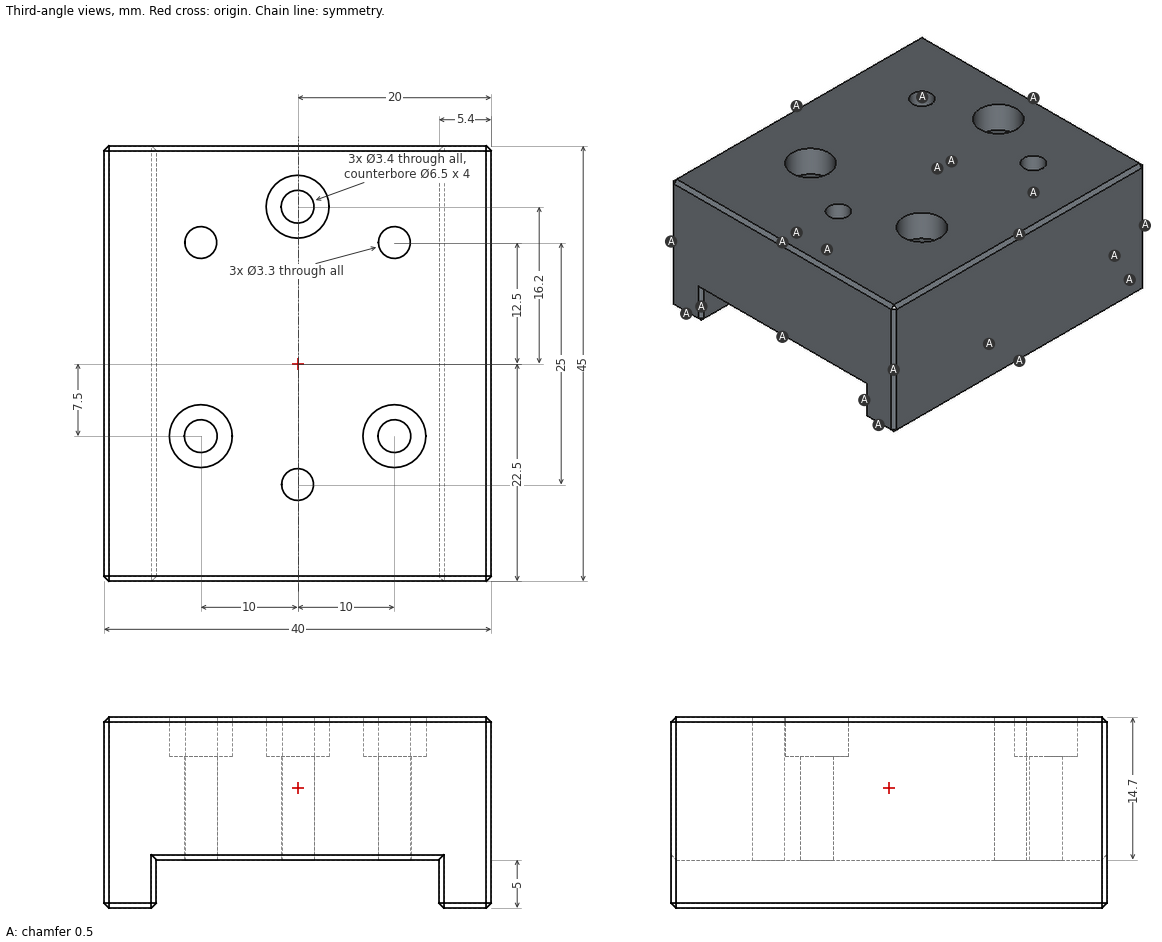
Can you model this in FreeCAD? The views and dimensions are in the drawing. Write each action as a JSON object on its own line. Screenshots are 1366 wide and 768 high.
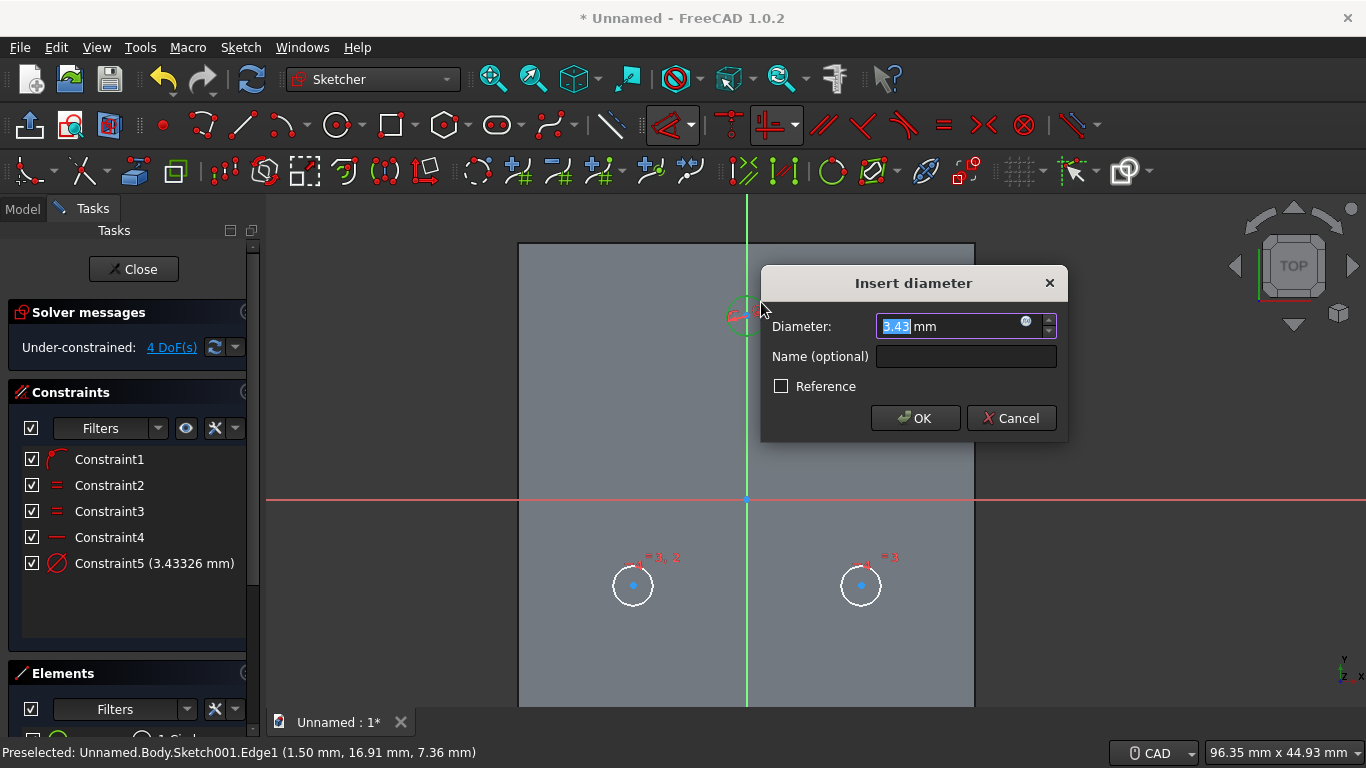
{"action": "type", "text": "3.4"}
{"action": "key", "text": "Return"}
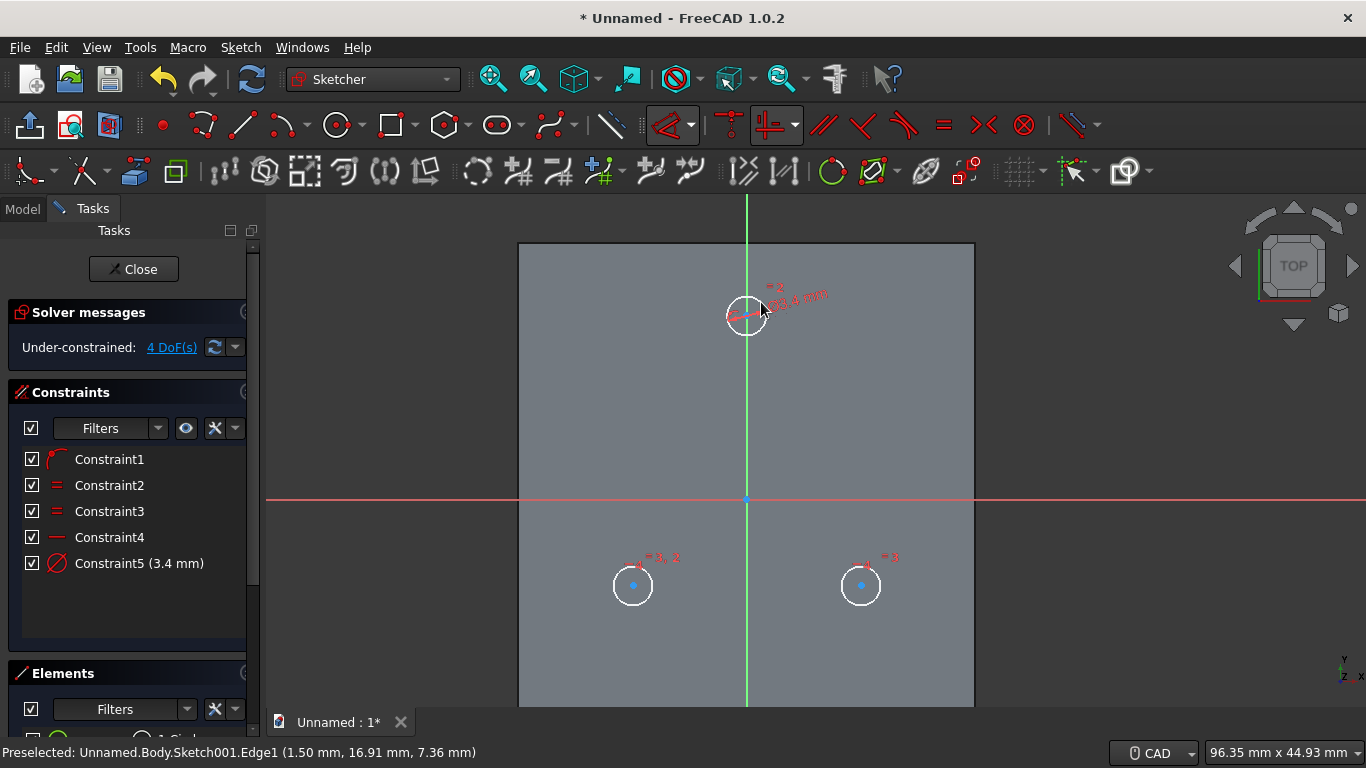
{"action": "left_click", "coordinate": [633, 586]}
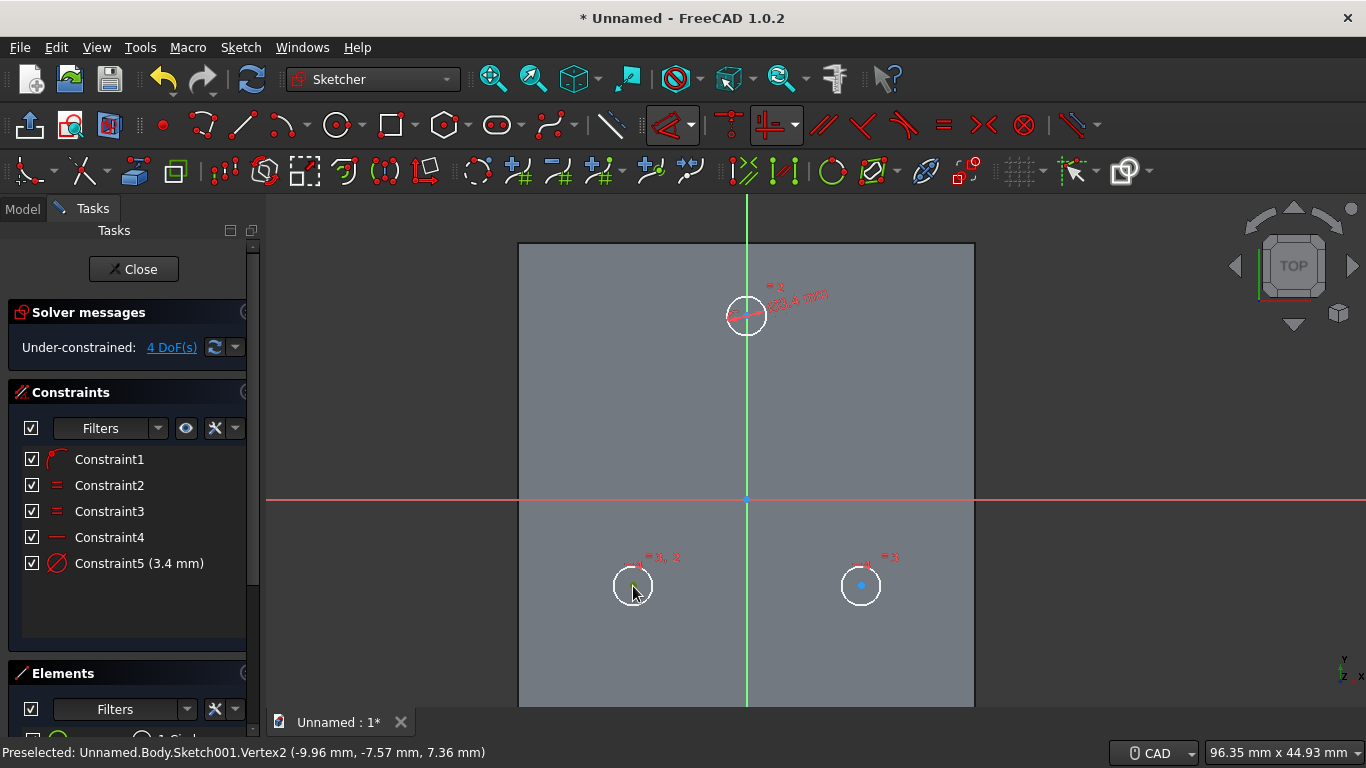
{"action": "key", "text": "l"}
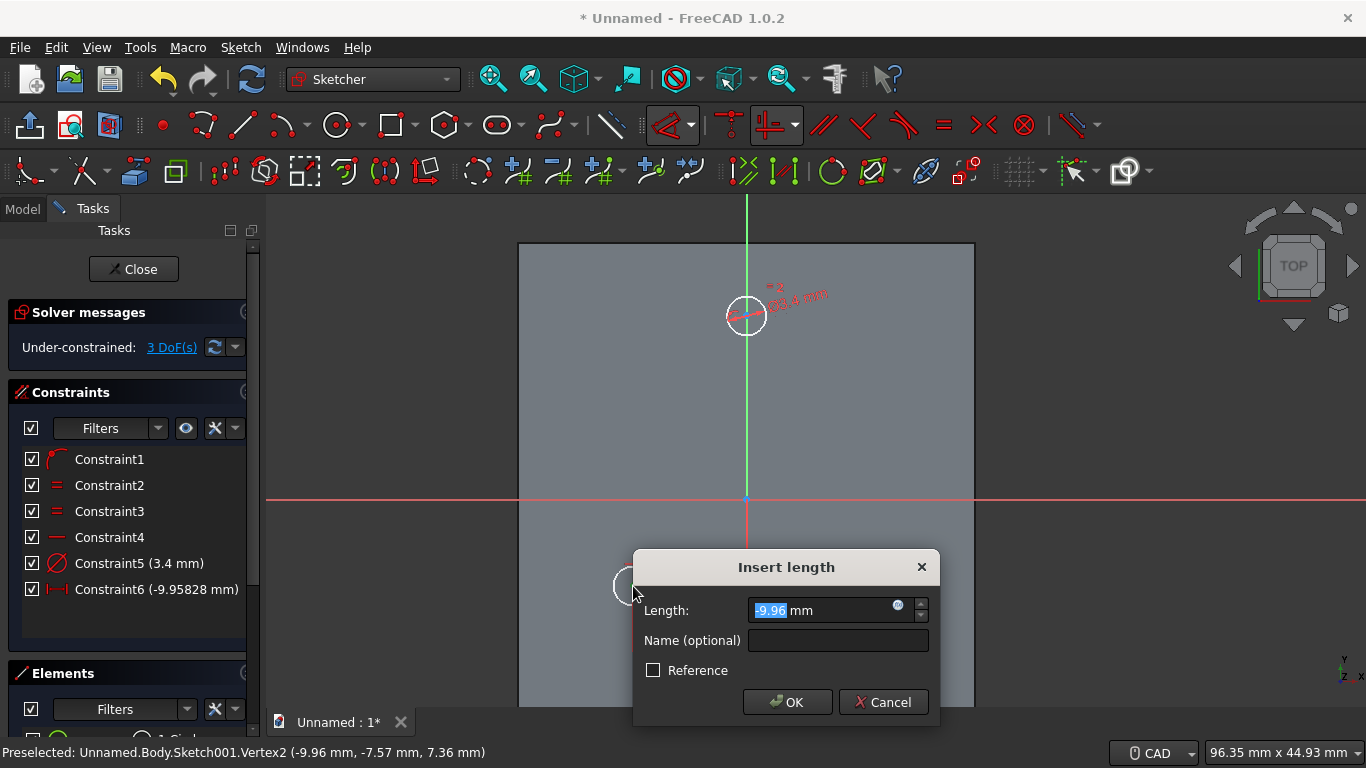
{"action": "type", "text": "-10"}
{"action": "key", "text": "Return"}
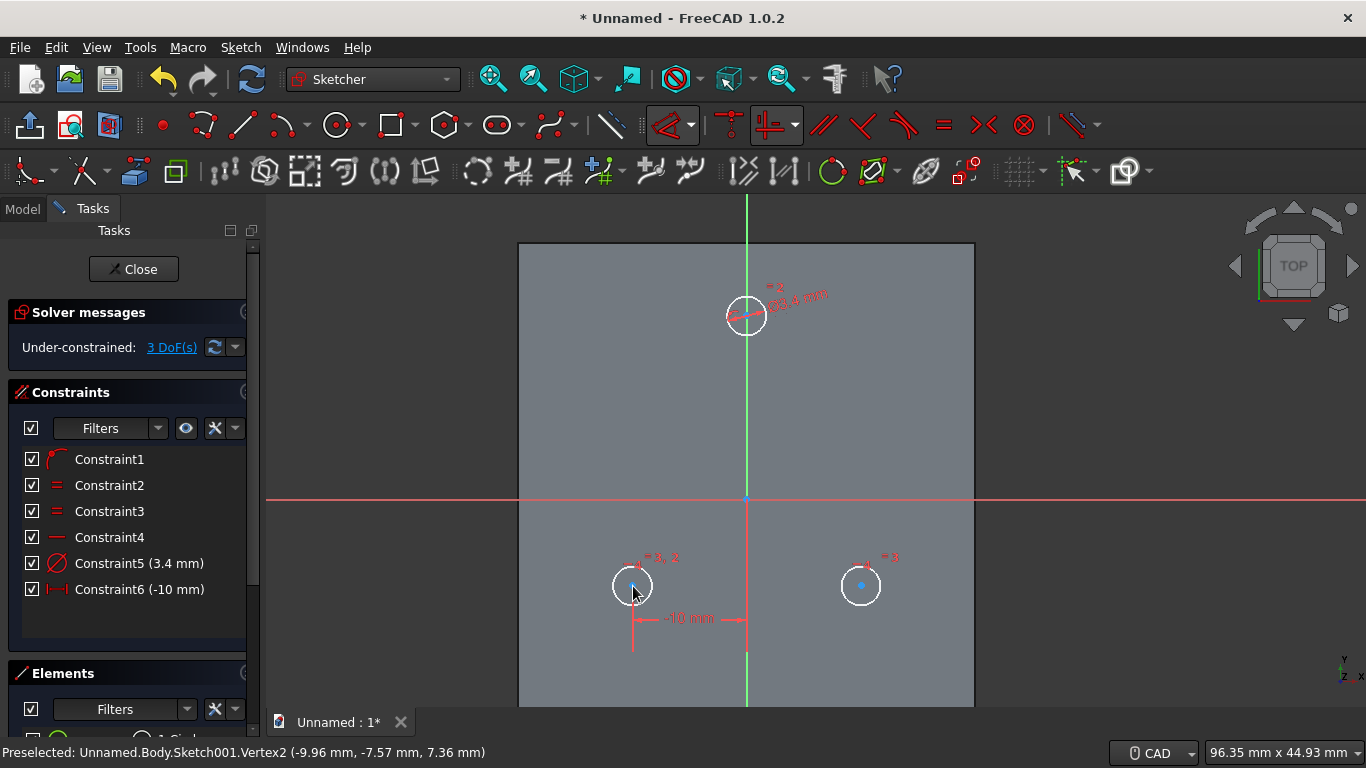
{"action": "left_click", "coordinate": [861, 586]}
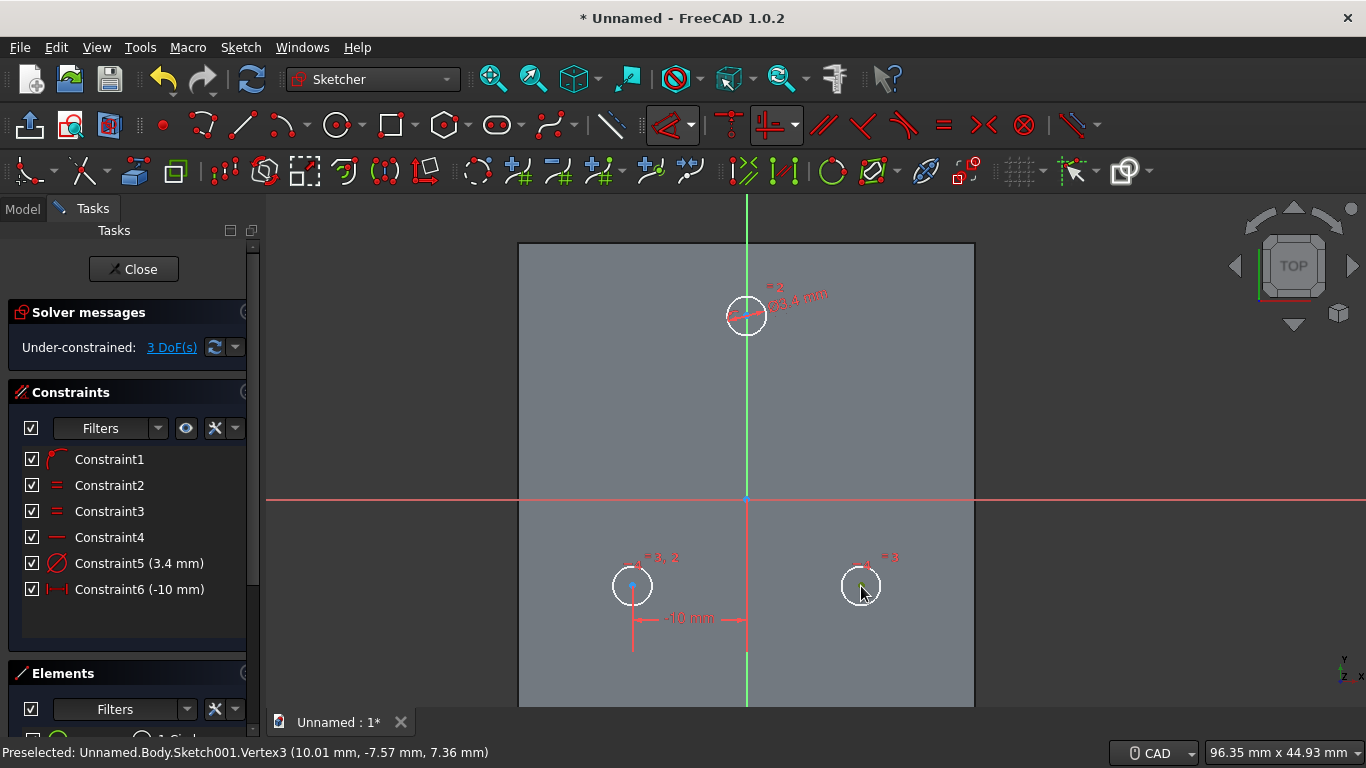
{"action": "left_click", "coordinate": [694, 126]}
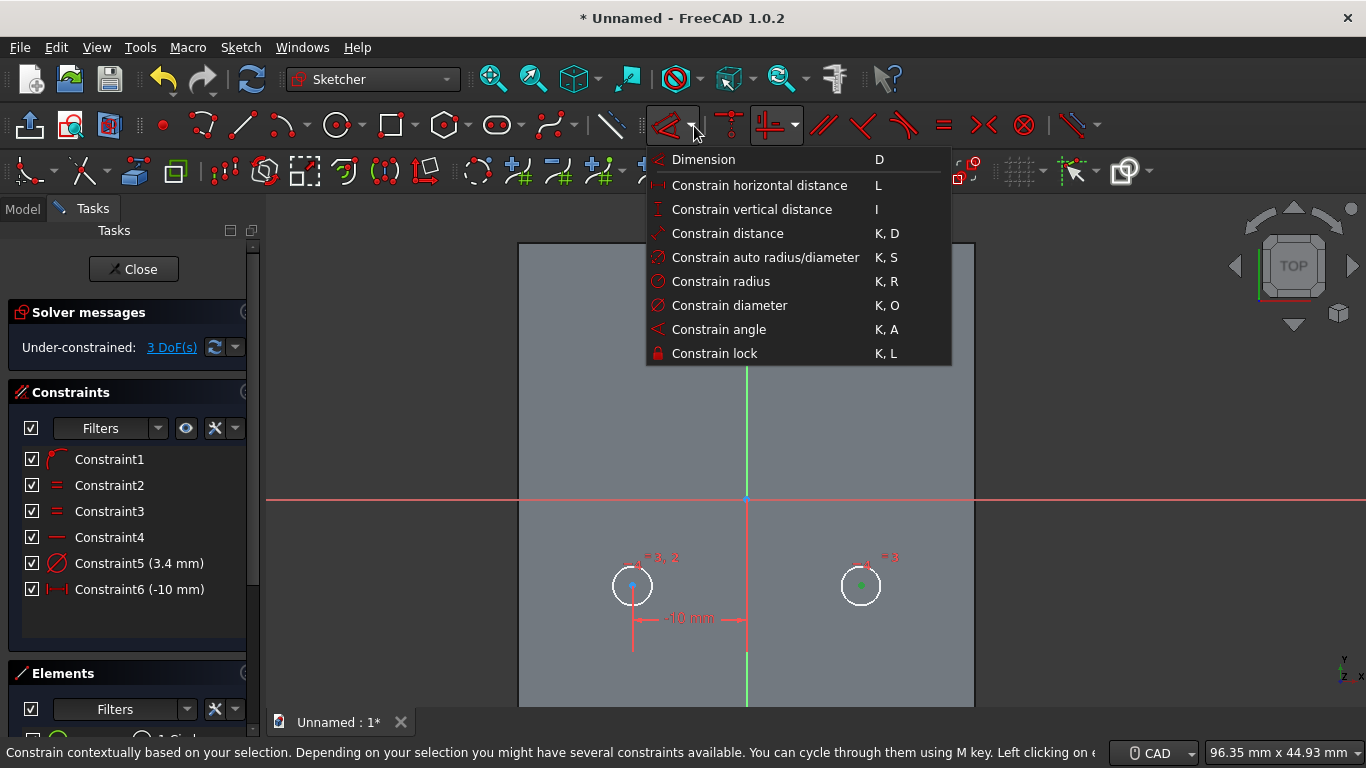
{"action": "left_click", "coordinate": [799, 185]}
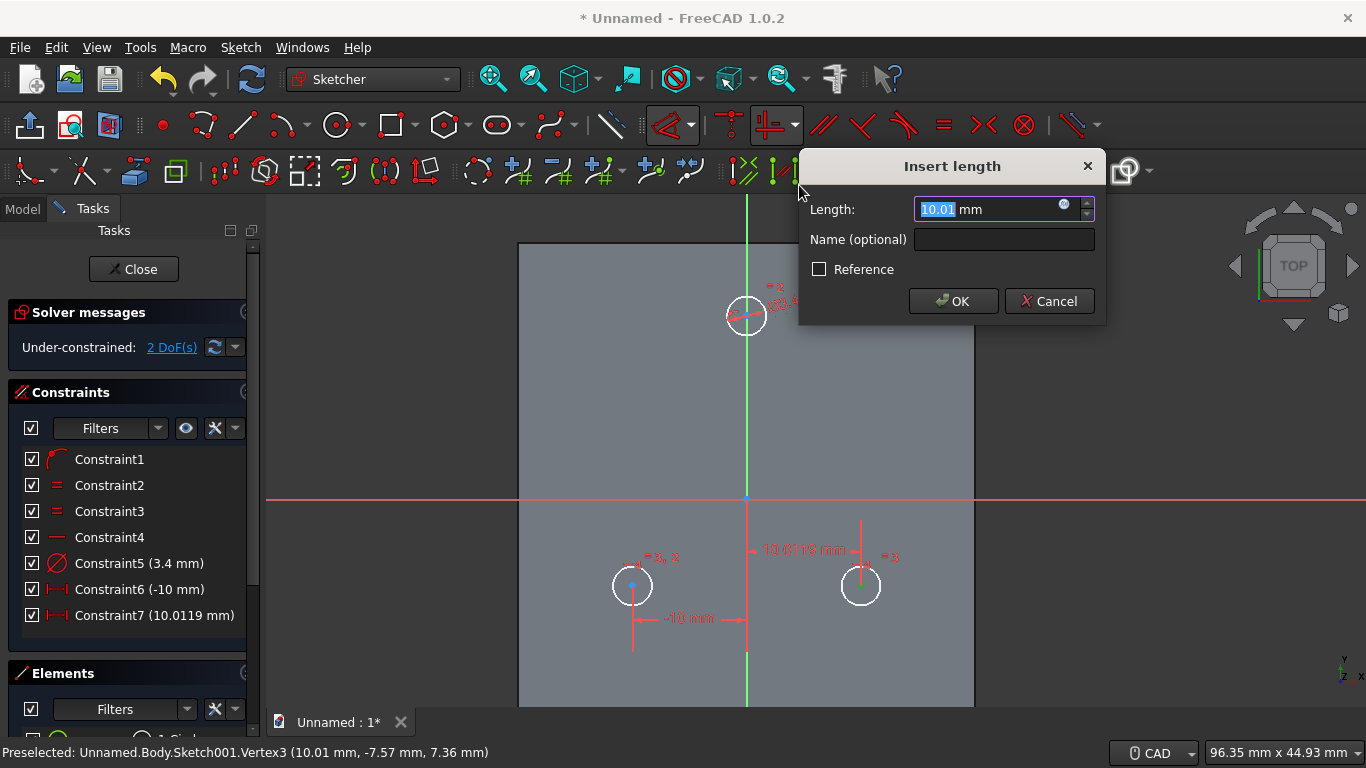
{"action": "type", "text": "10"}
{"action": "key", "text": "Return"}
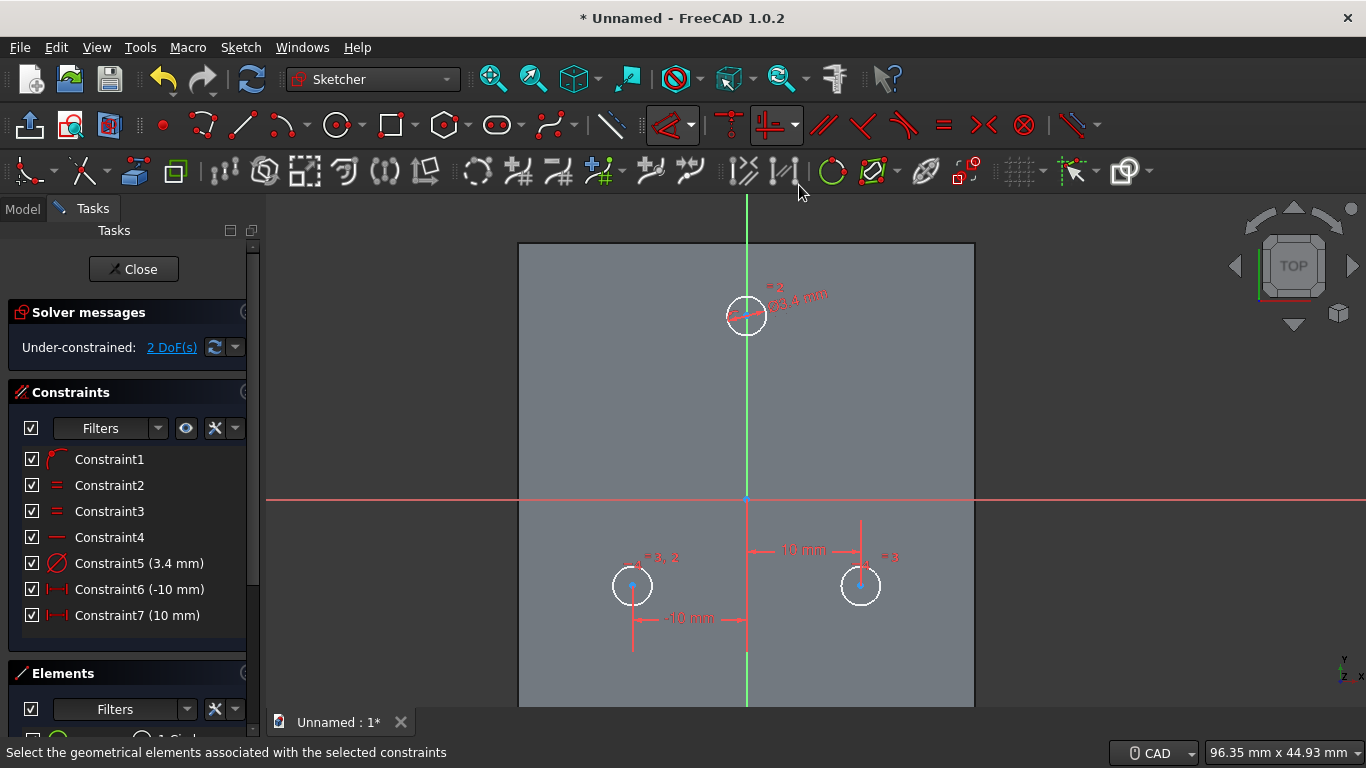
{"action": "left_click", "coordinate": [633, 586]}